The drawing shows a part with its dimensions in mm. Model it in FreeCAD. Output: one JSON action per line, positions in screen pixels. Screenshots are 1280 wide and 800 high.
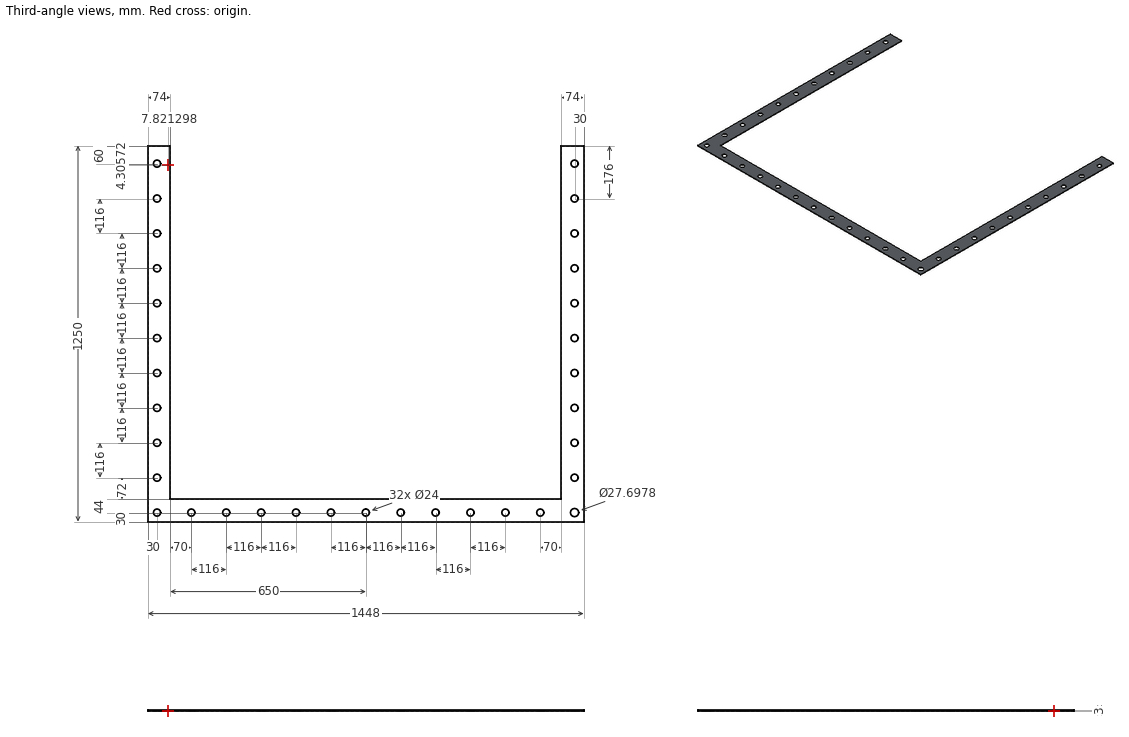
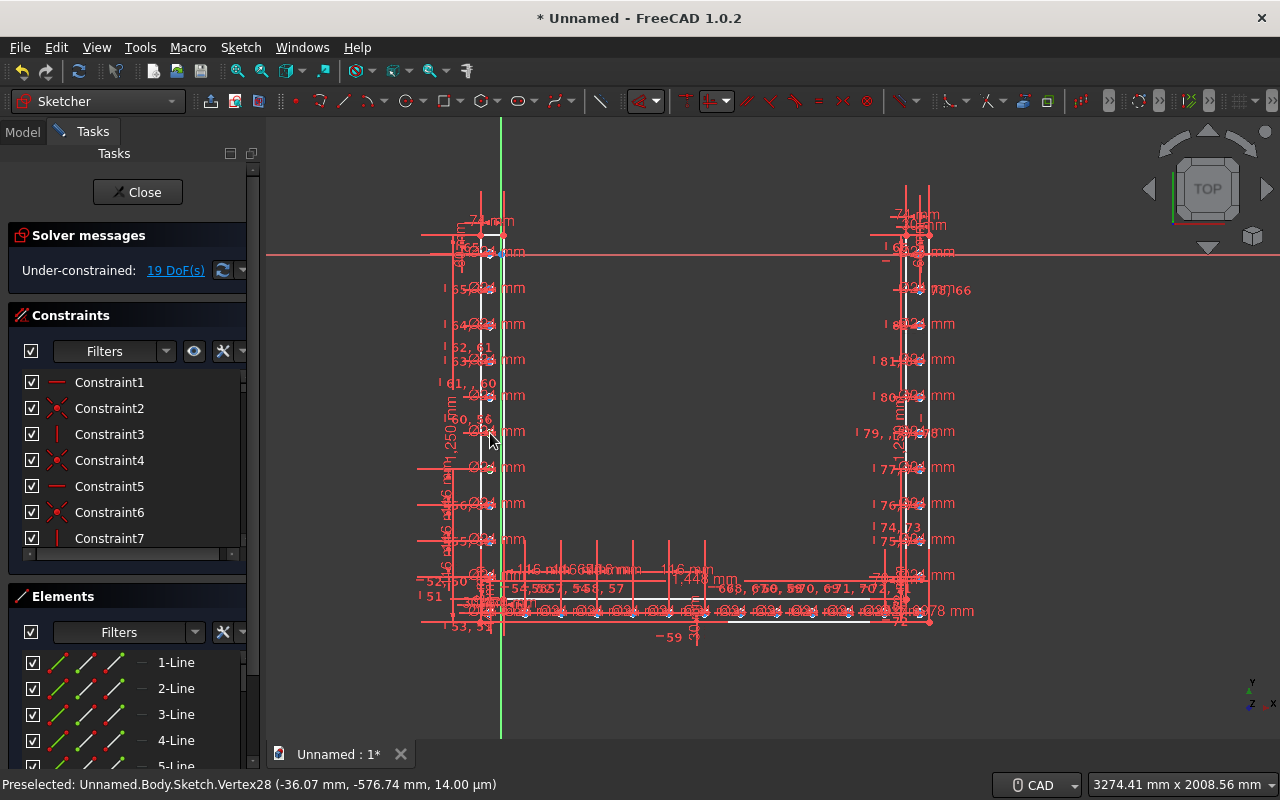
{"action": "left_click", "coordinate": [658, 102]}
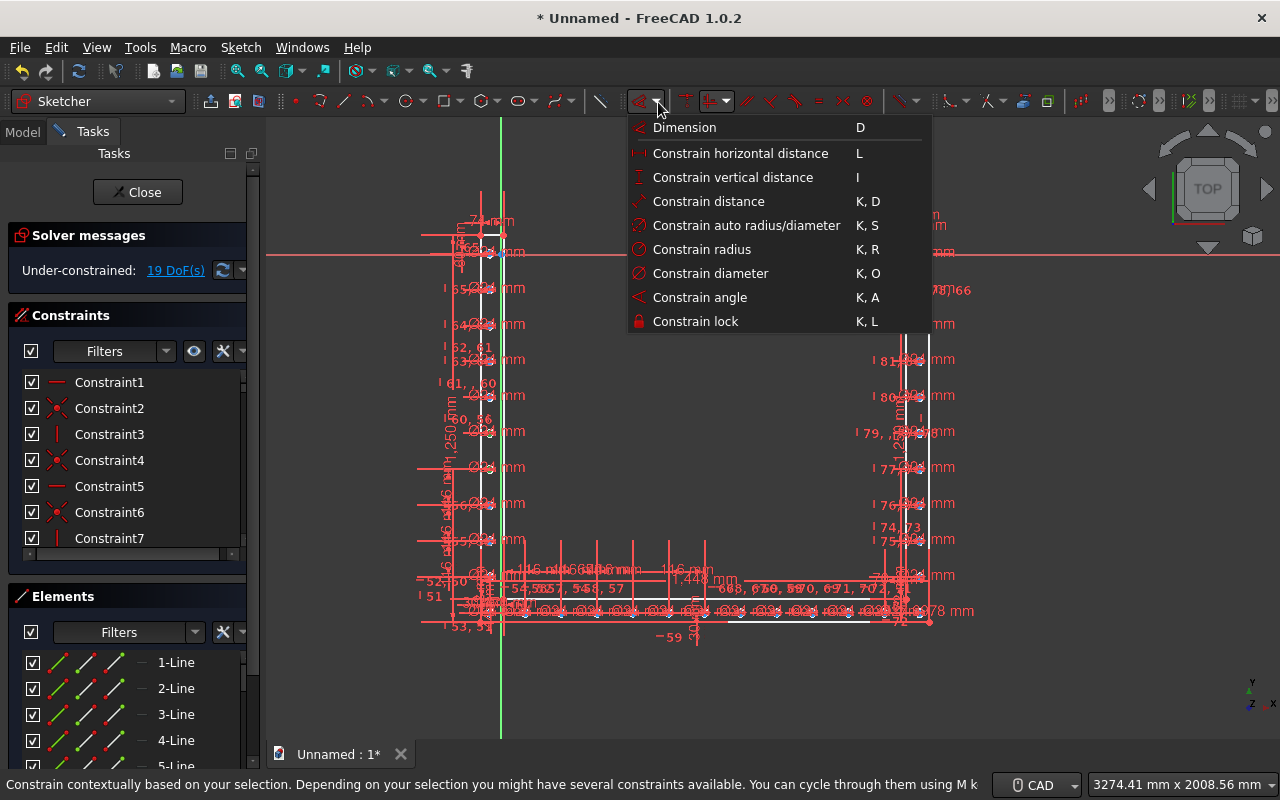
{"action": "left_click", "coordinate": [780, 177]}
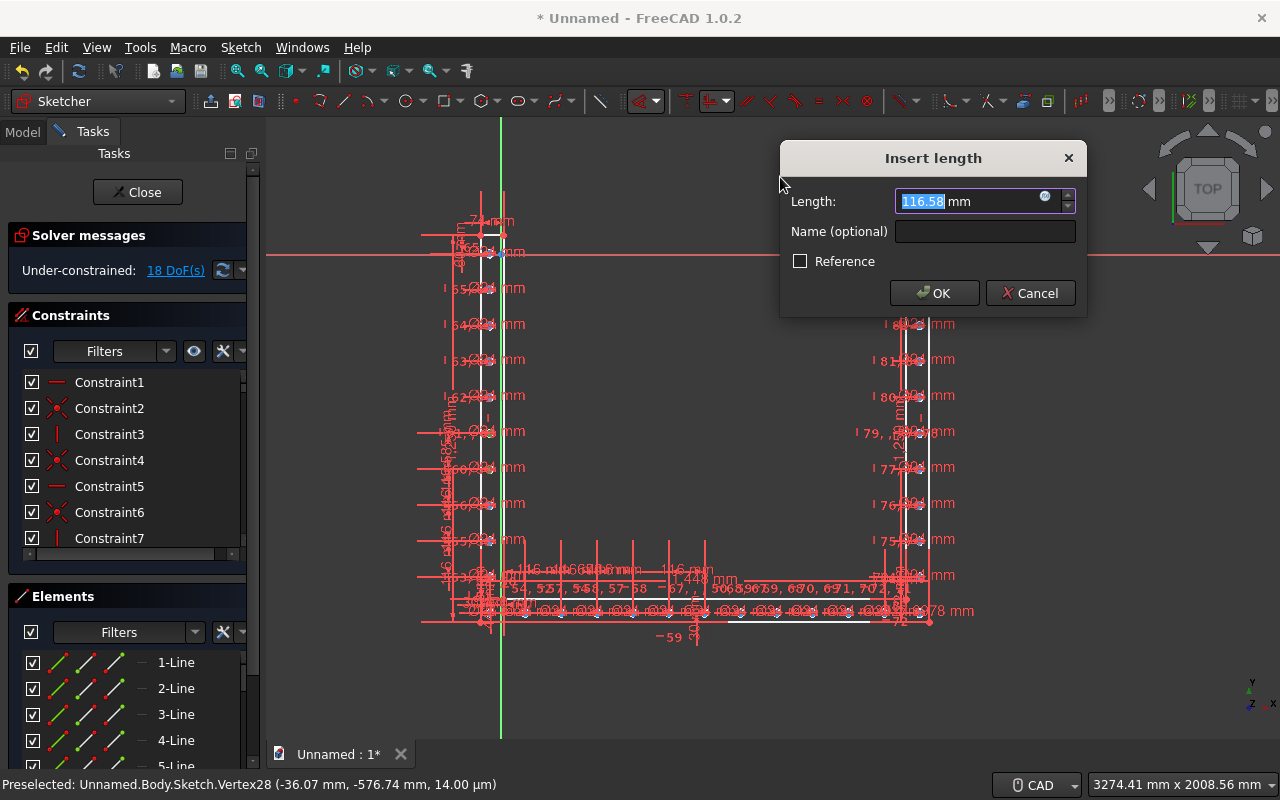
{"action": "type", "text": "116"}
{"action": "key", "text": "Return"}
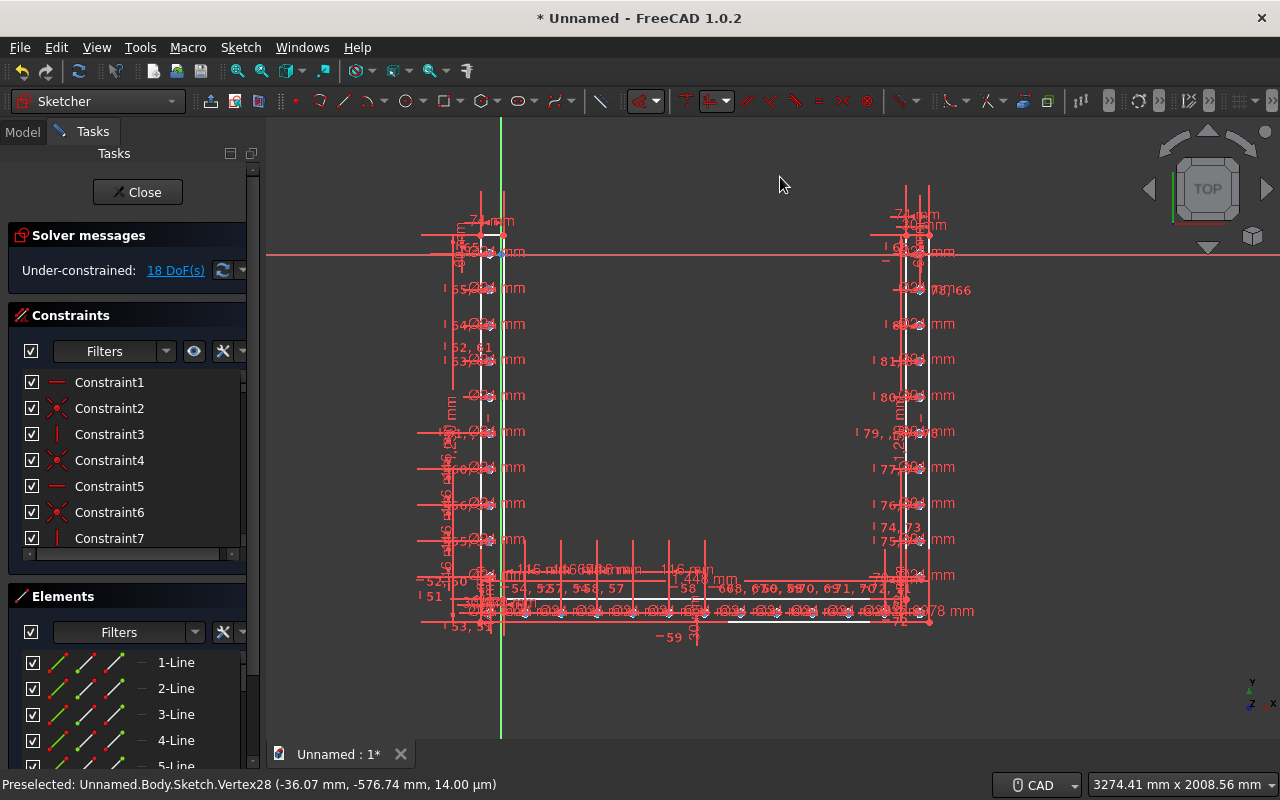
{"action": "left_click", "coordinate": [490, 433]}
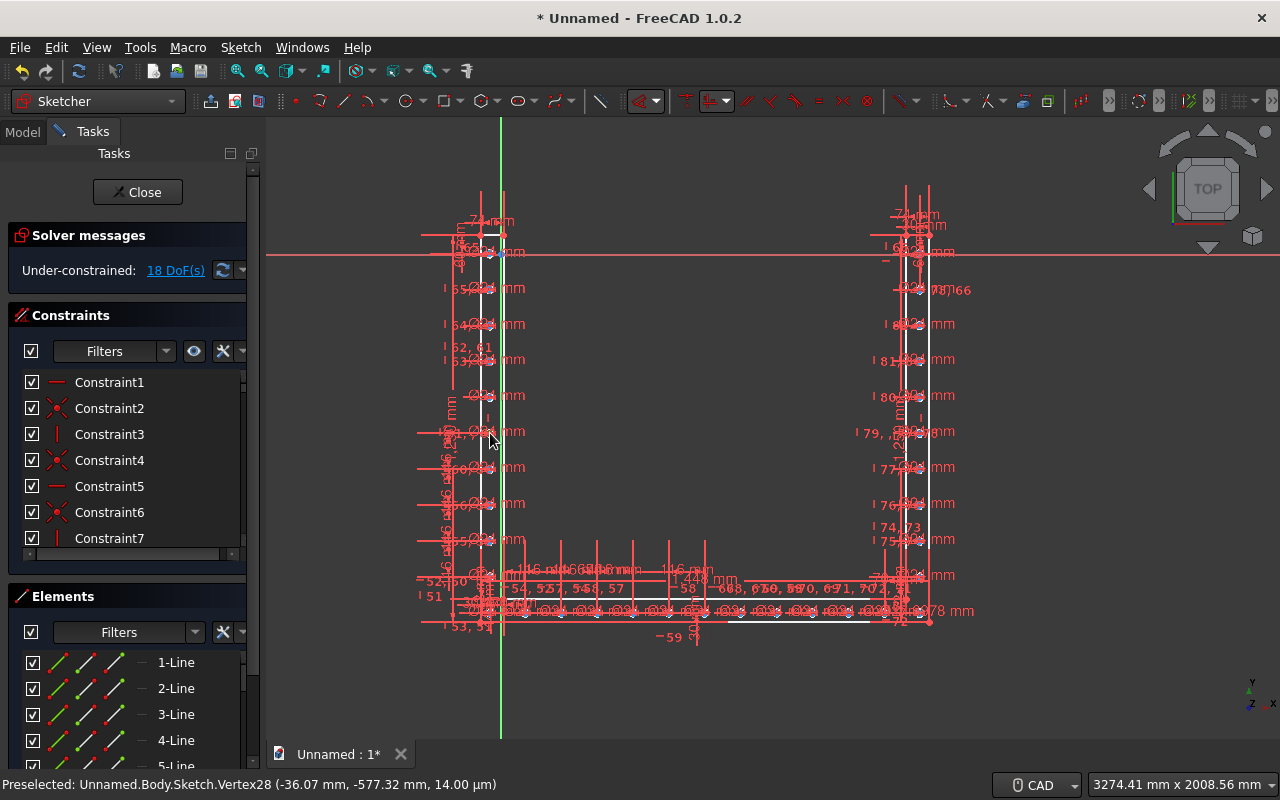
{"action": "left_click", "coordinate": [490, 397]}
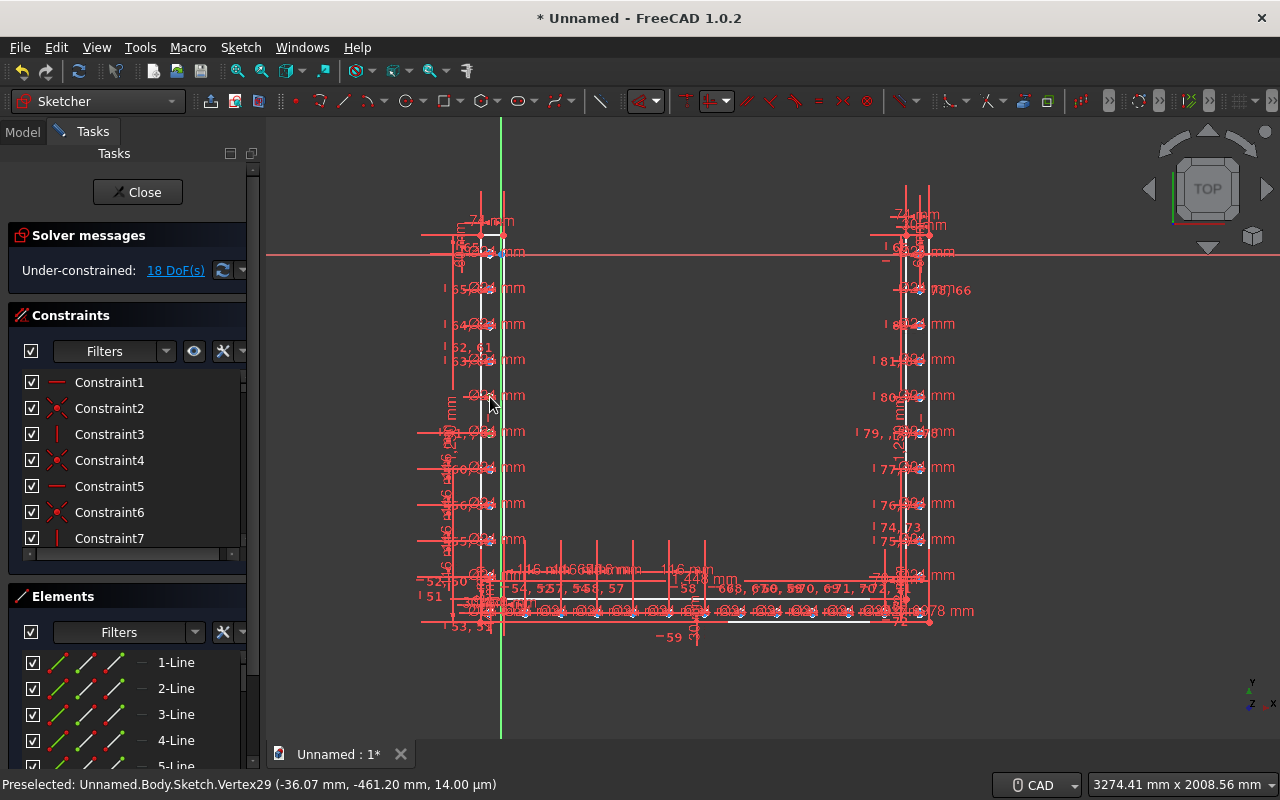
{"action": "left_click", "coordinate": [658, 102]}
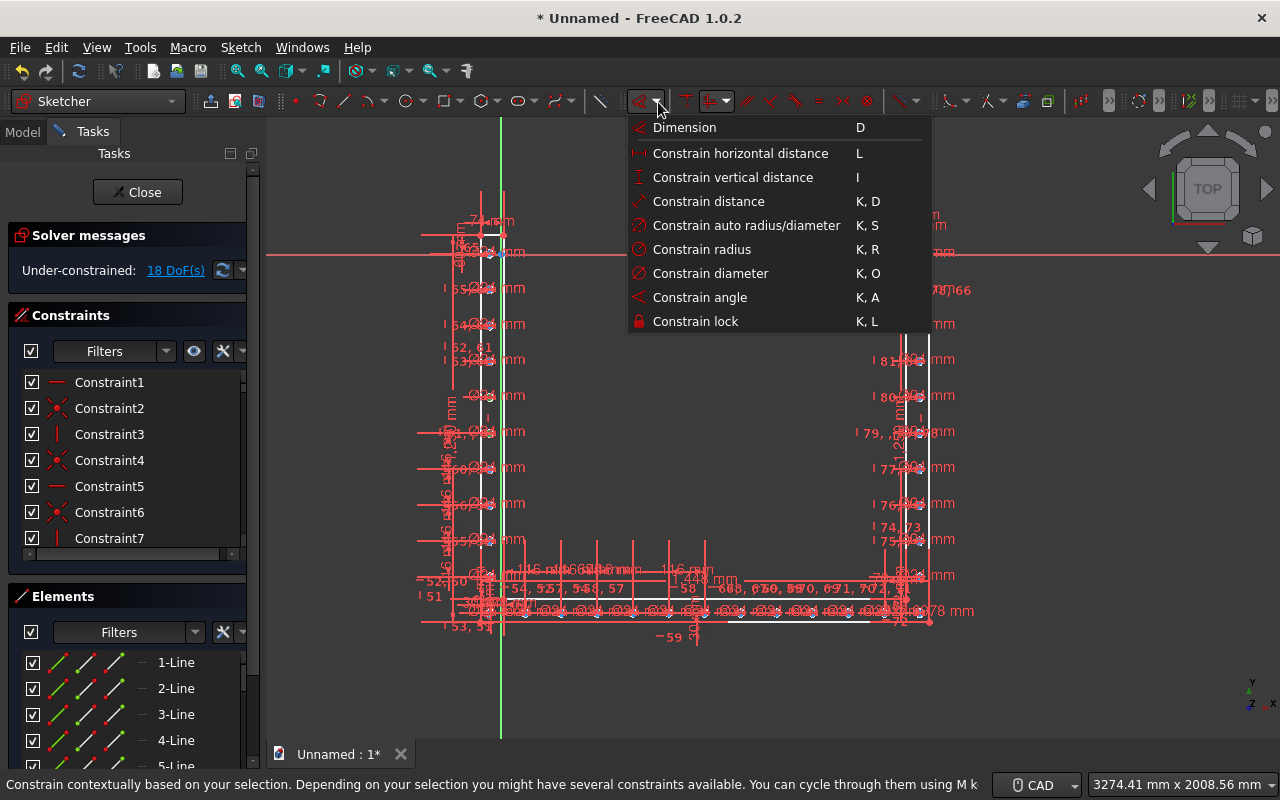
{"action": "left_click", "coordinate": [780, 177]}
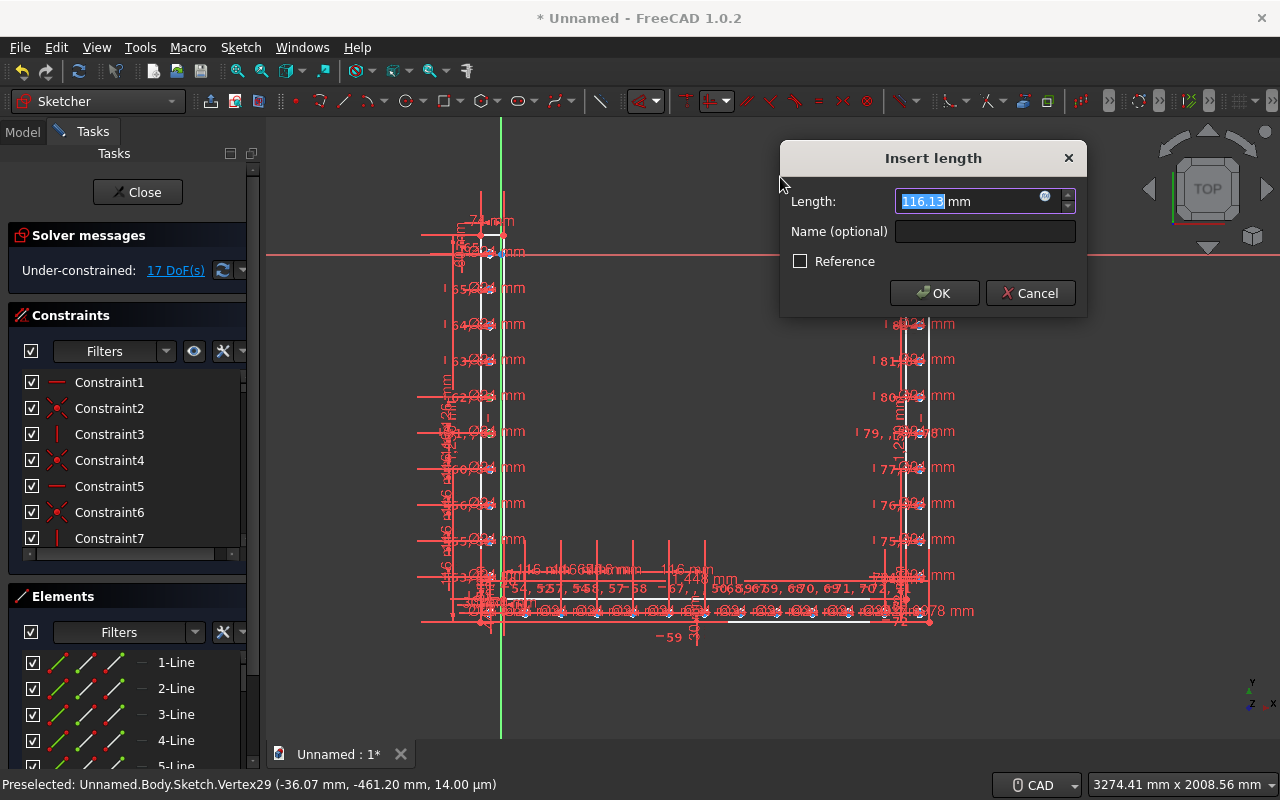
{"action": "type", "text": "116"}
{"action": "key", "text": "Return"}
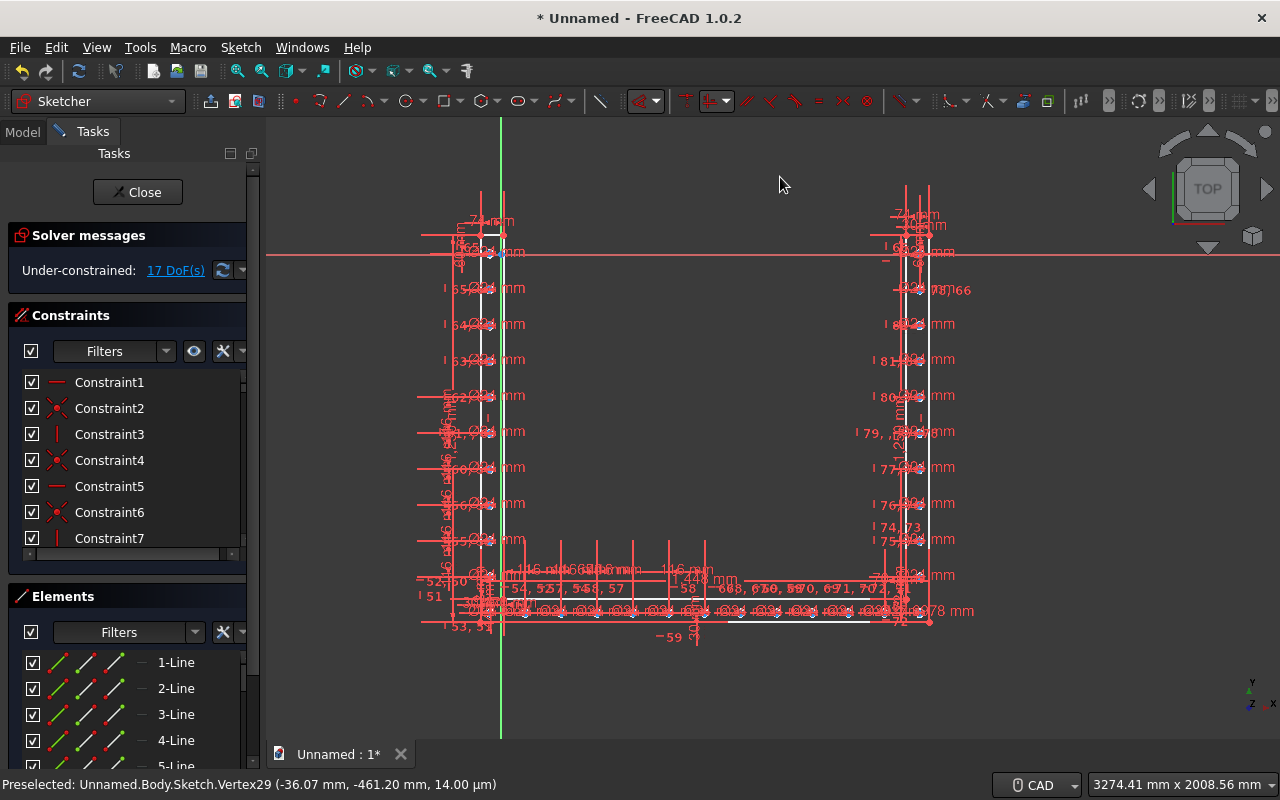
{"action": "left_click", "coordinate": [490, 397]}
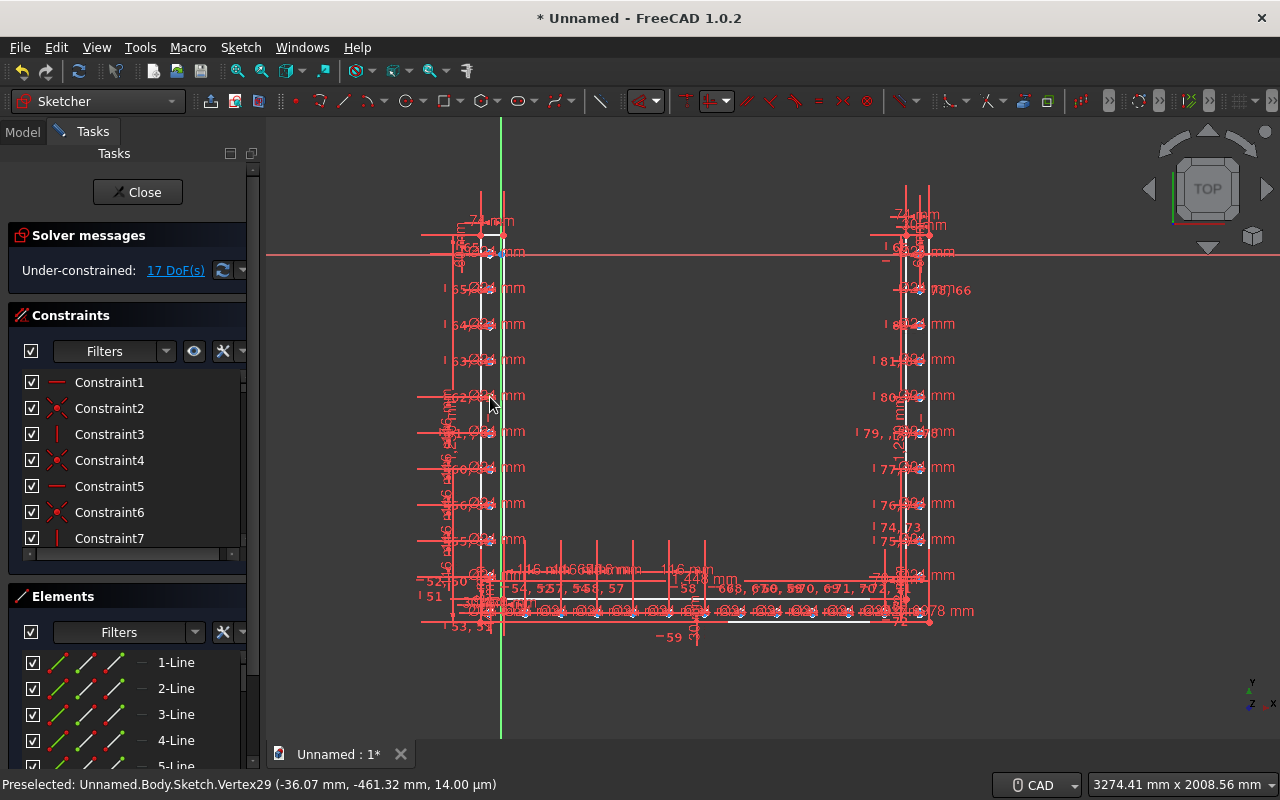
{"action": "left_click", "coordinate": [490, 361]}